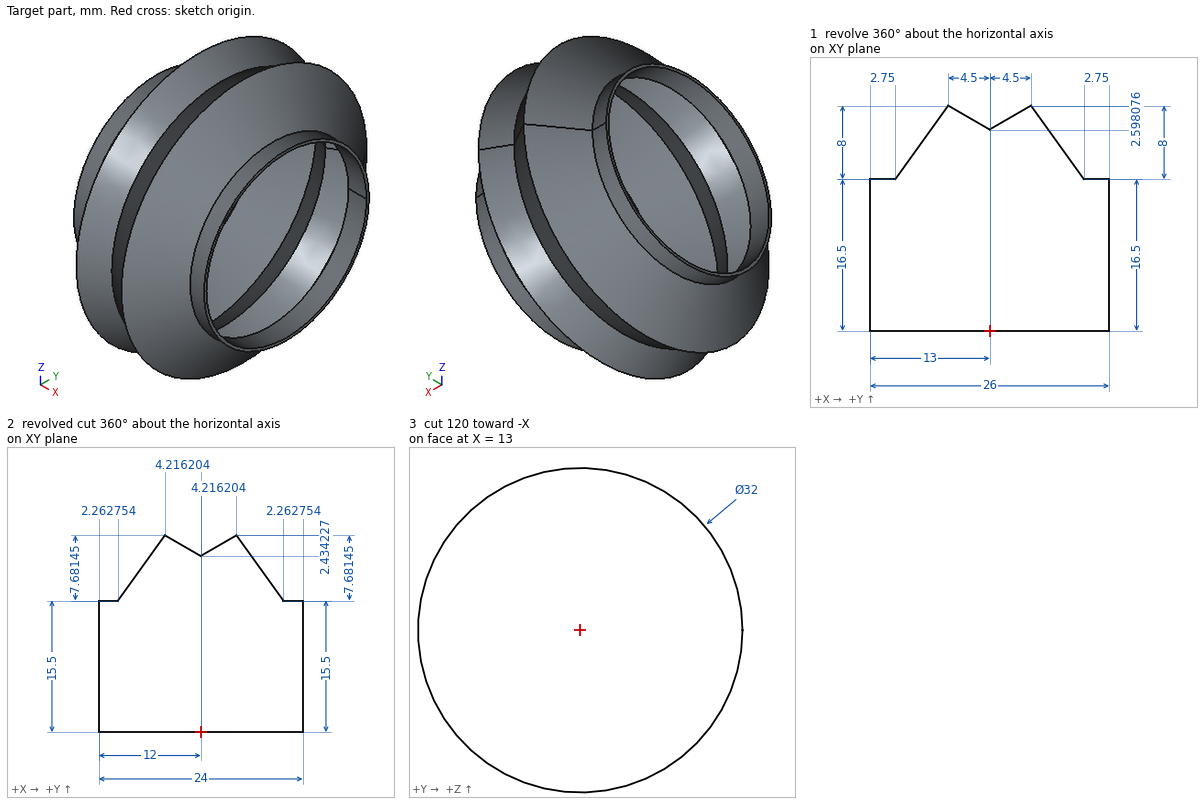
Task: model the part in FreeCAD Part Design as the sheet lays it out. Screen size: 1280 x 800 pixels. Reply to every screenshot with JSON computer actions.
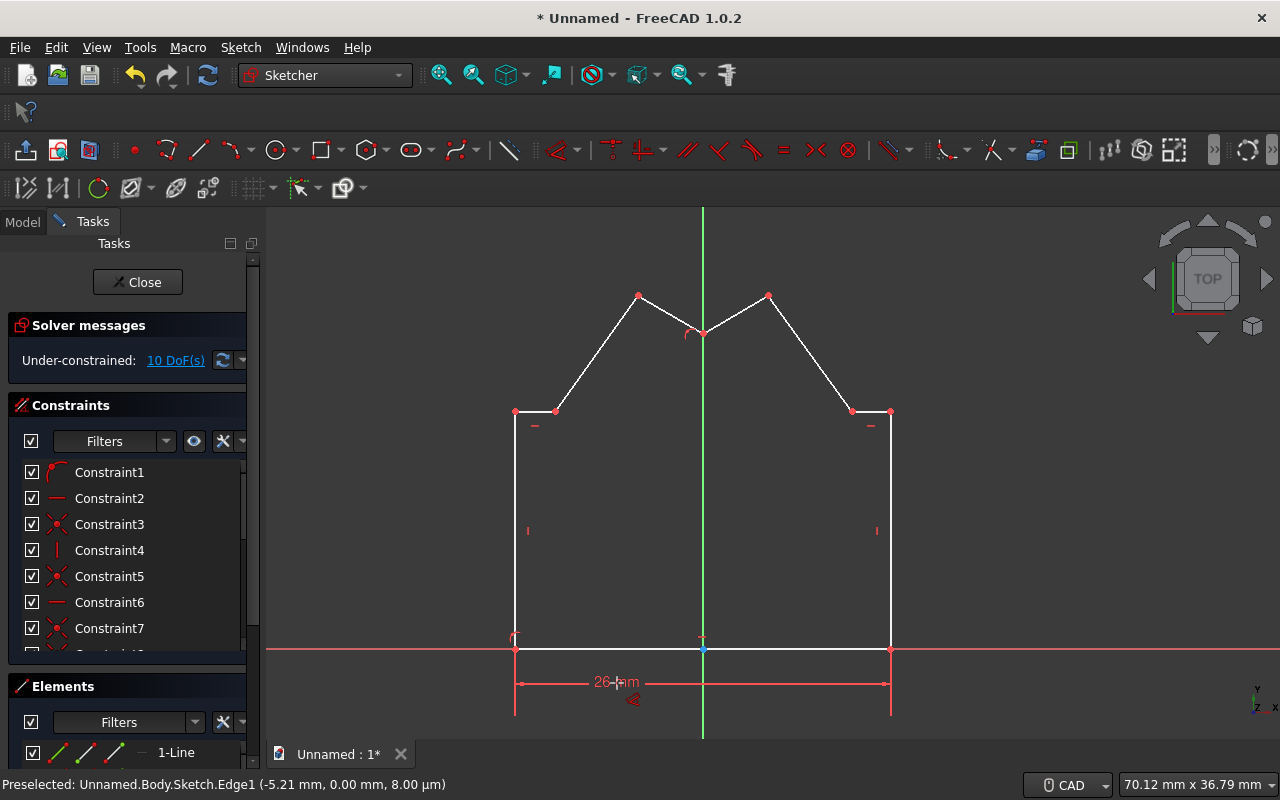
{"action": "left_click", "coordinate": [827, 377]}
{"action": "left_click", "coordinate": [886, 354]}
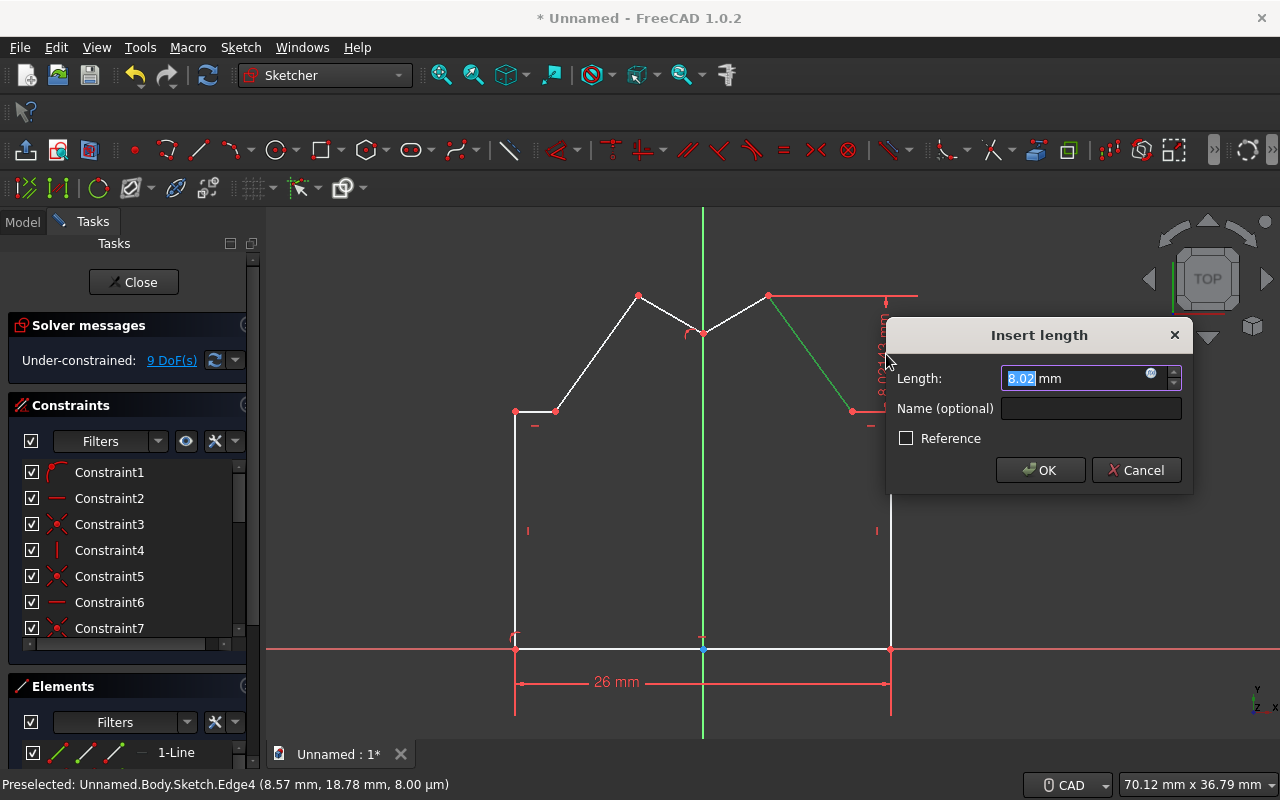
{"action": "type", "text": "8"}
{"action": "key", "text": "Return"}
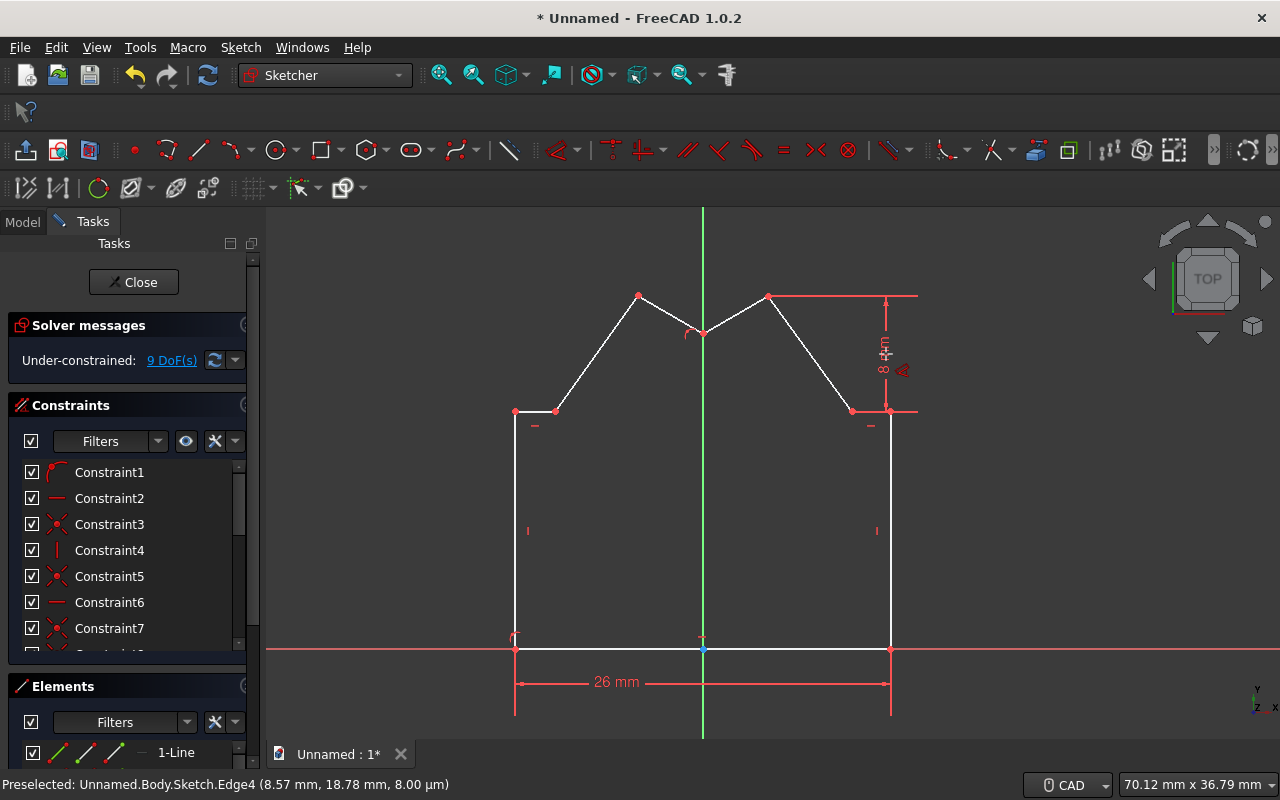
{"action": "left_click", "coordinate": [613, 331]}
{"action": "left_click", "coordinate": [521, 354]}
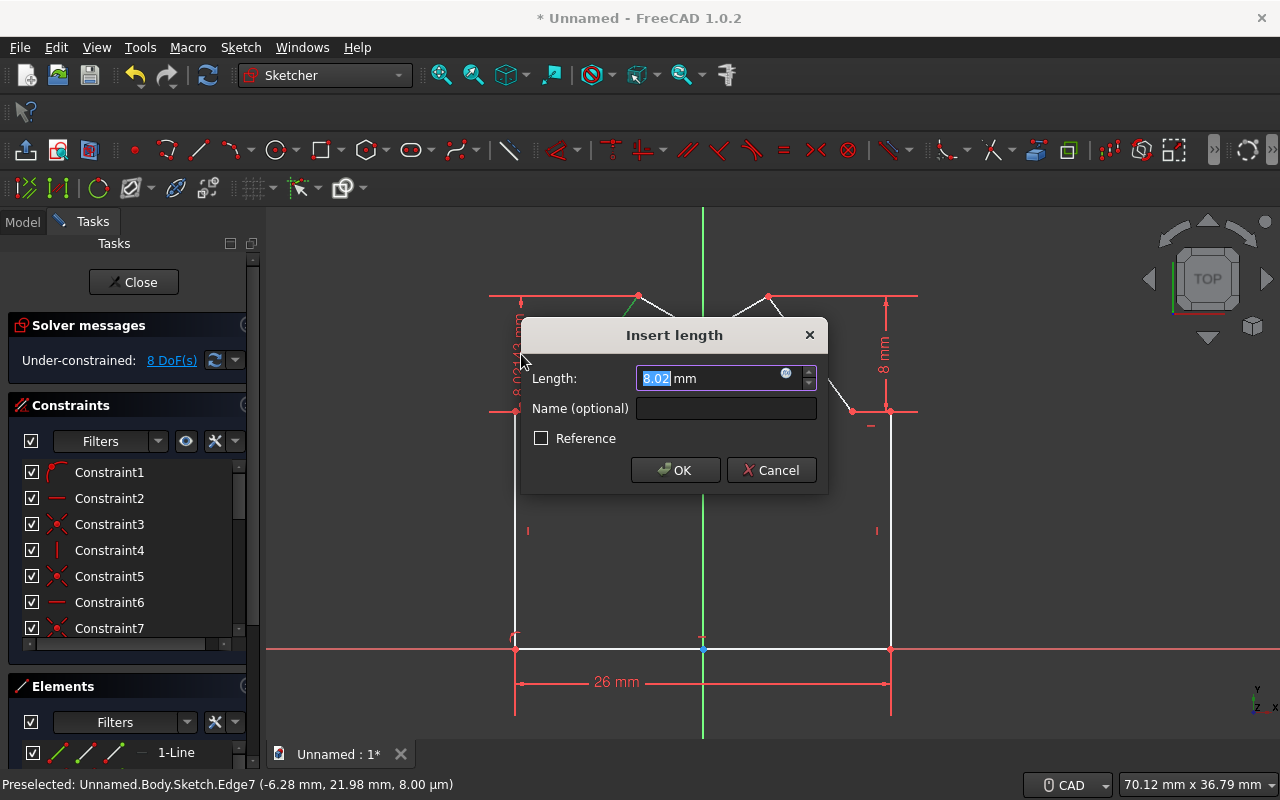
{"action": "type", "text": "8"}
{"action": "key", "text": "Return"}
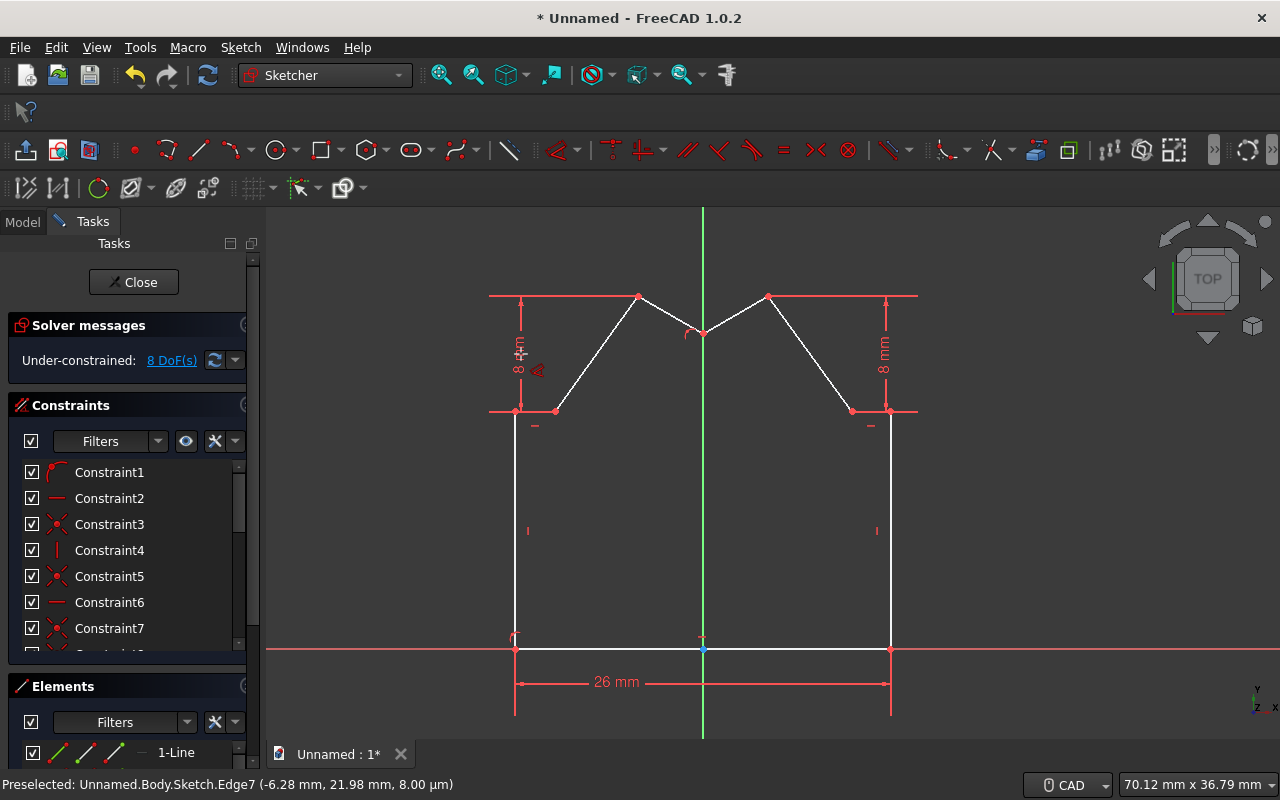
{"action": "left_click", "coordinate": [515, 649]}
{"action": "left_click", "coordinate": [543, 683]}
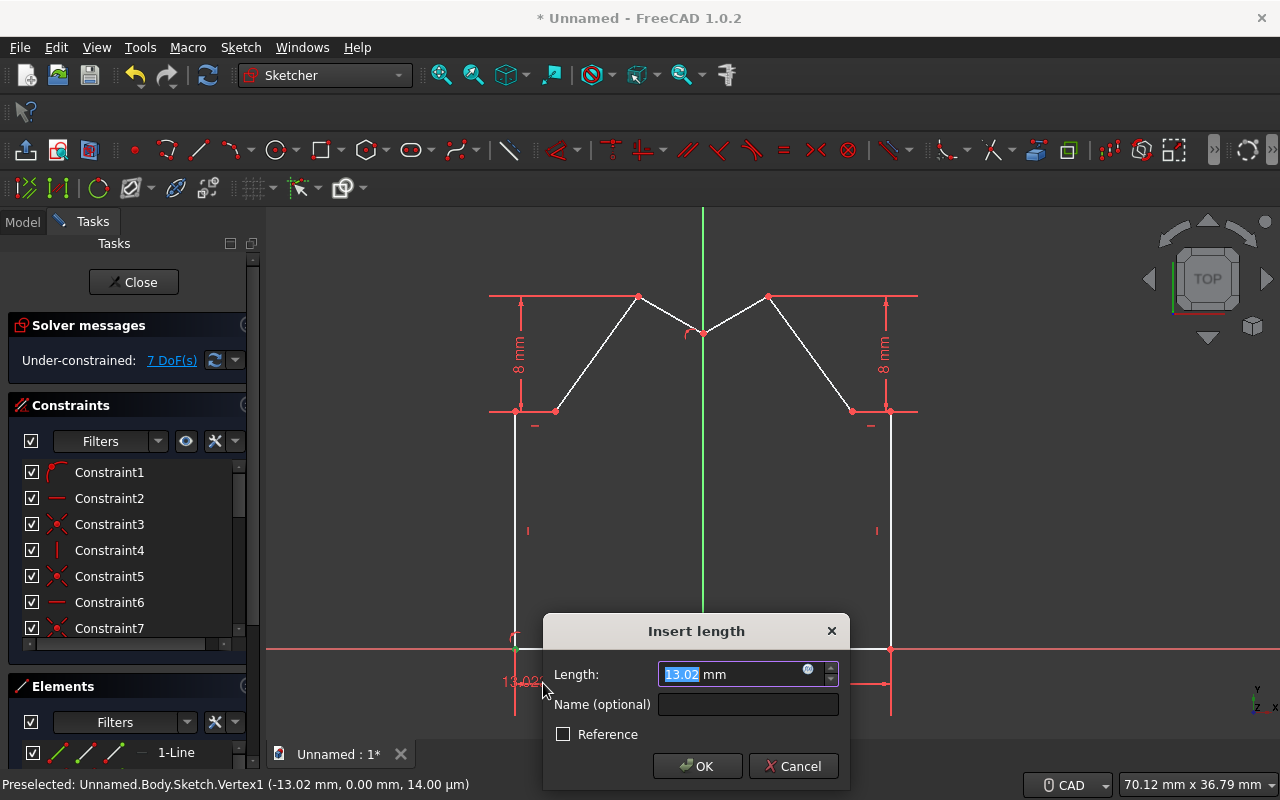
{"action": "type", "text": "13"}
{"action": "key", "text": "Return"}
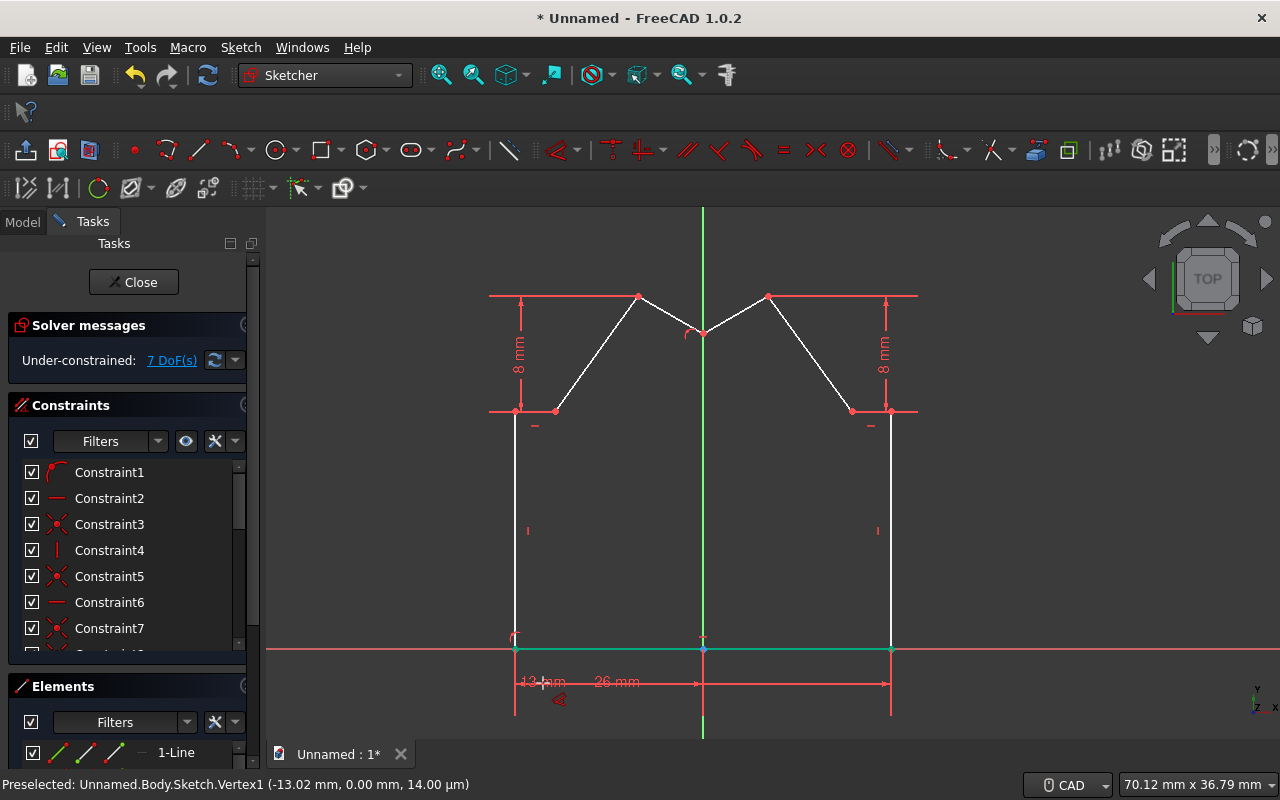
{"action": "left_click", "coordinate": [891, 578]}
{"action": "left_click", "coordinate": [925, 531]}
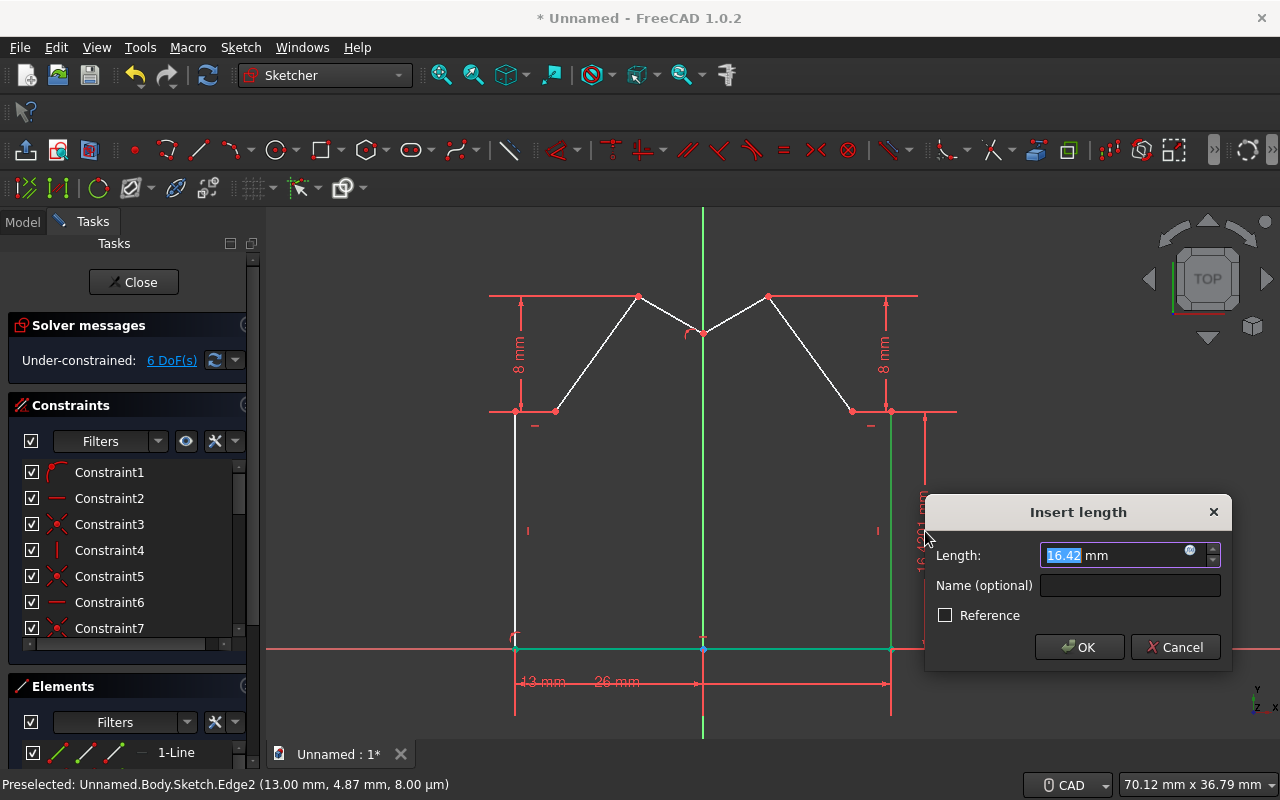
{"action": "type", "text": "16.5"}
{"action": "key", "text": "Return"}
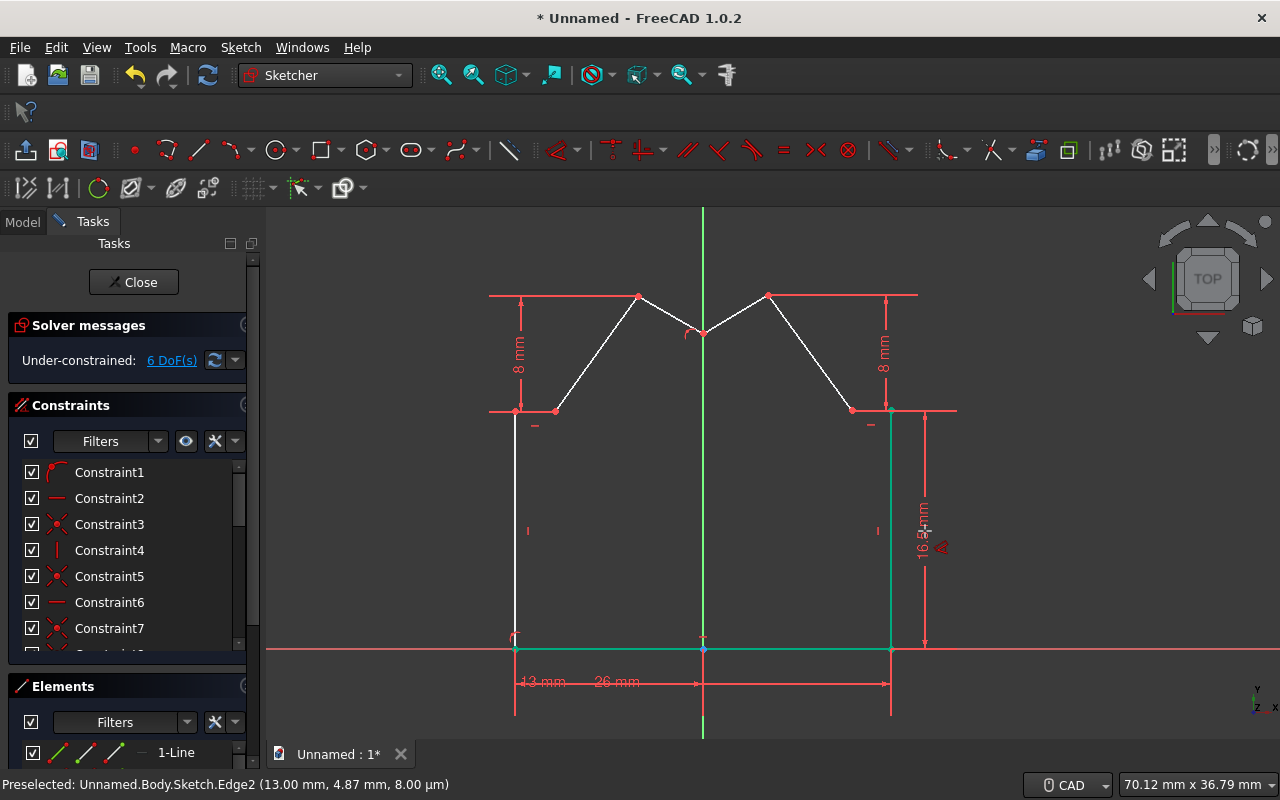
{"action": "left_click", "coordinate": [880, 411]}
{"action": "left_click", "coordinate": [872, 377]}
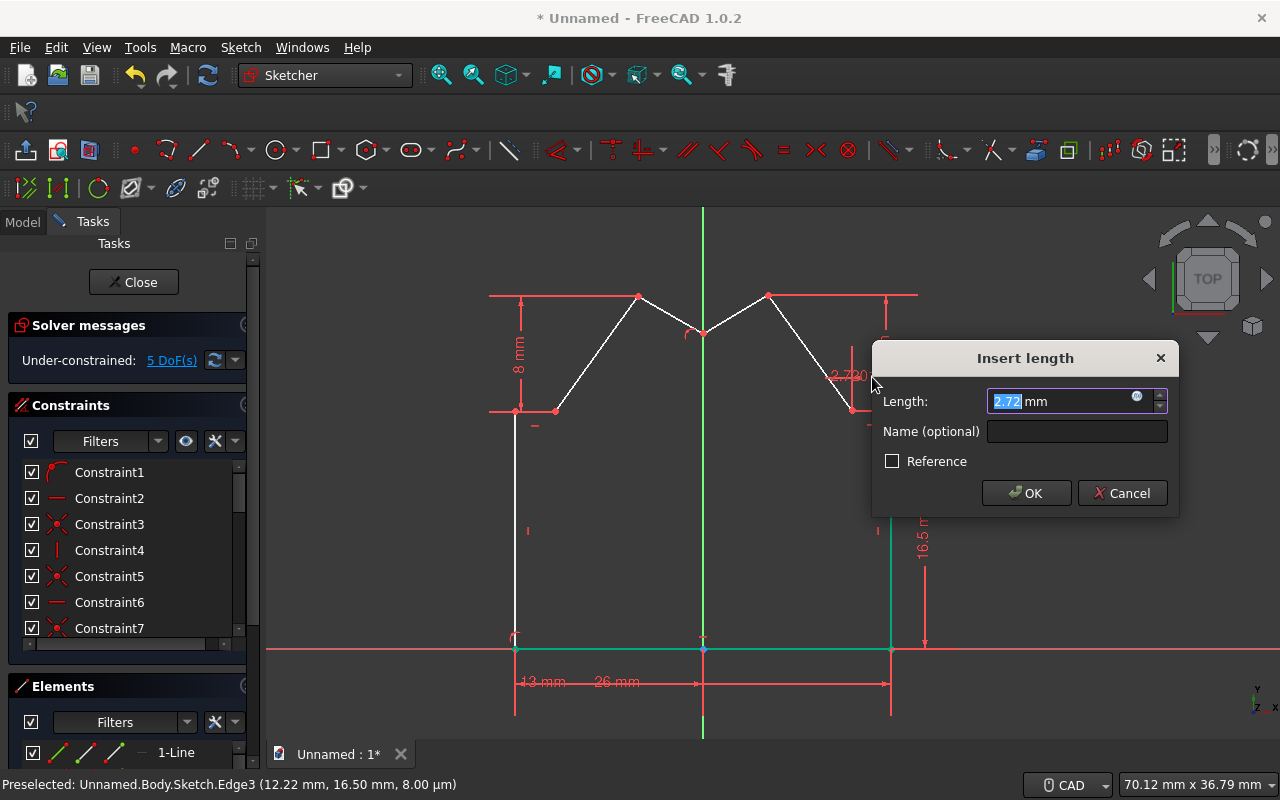
{"action": "type", "text": "2.75"}
{"action": "key", "text": "Return"}